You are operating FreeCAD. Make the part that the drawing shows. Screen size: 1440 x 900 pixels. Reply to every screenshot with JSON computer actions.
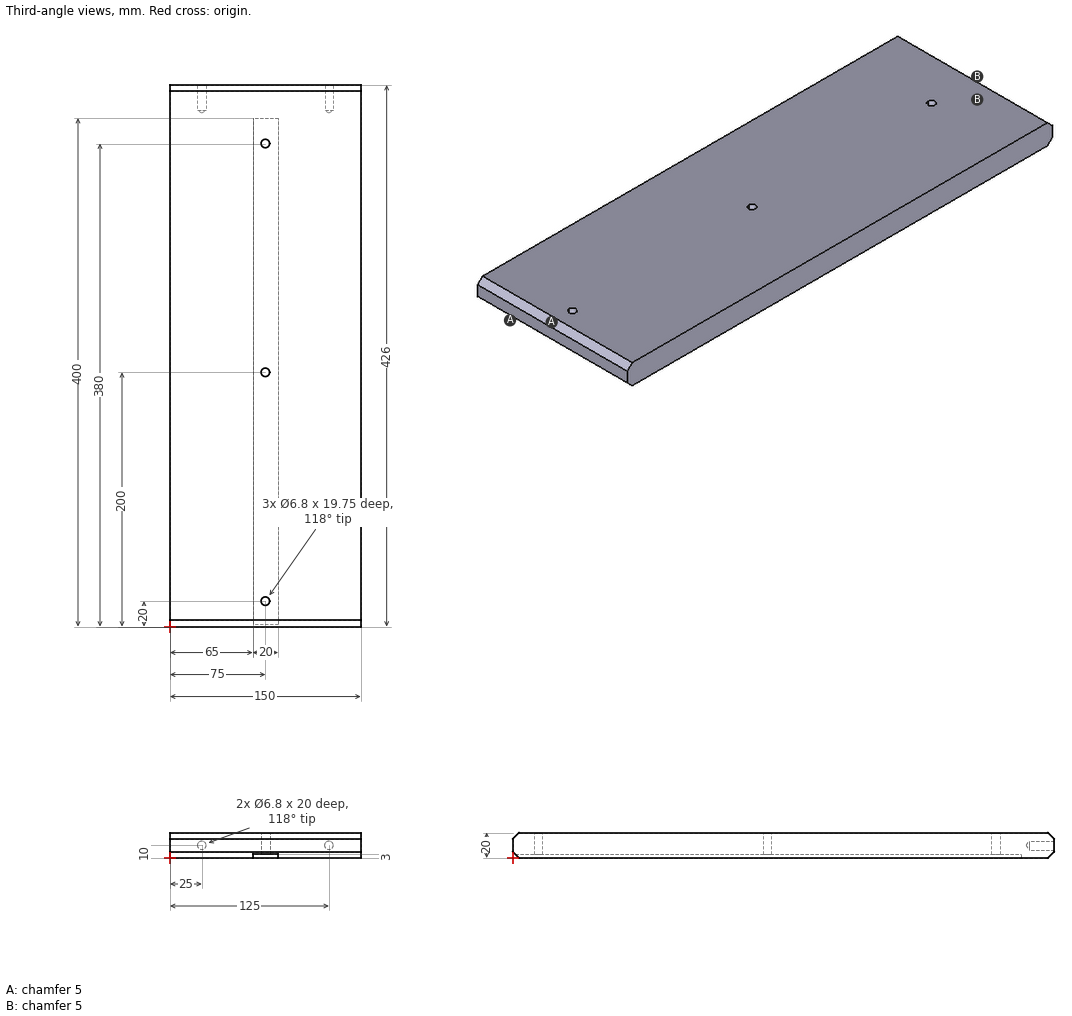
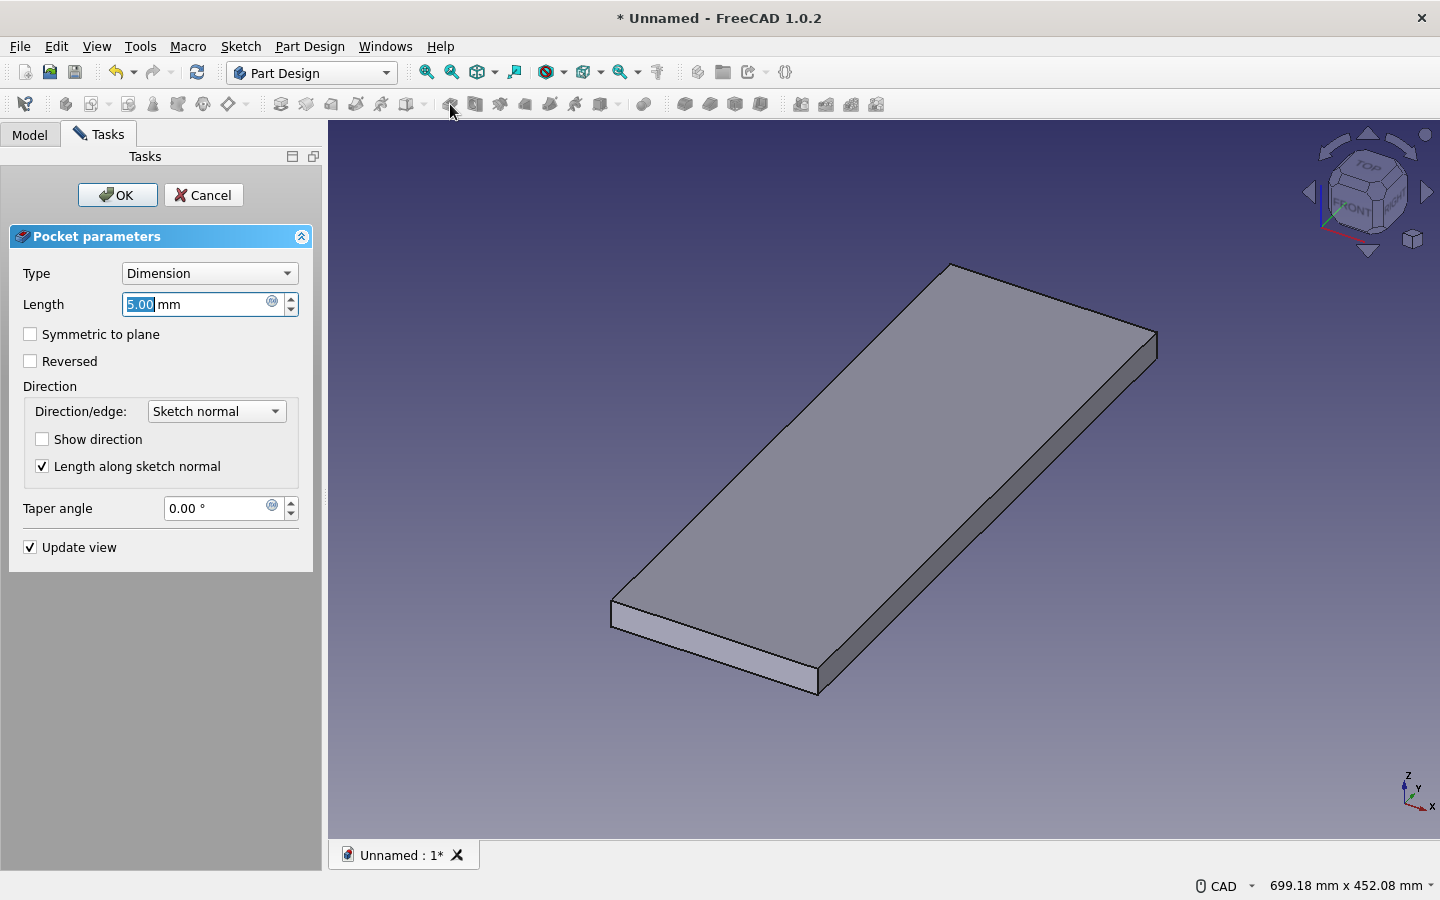
{"action": "type", "text": "3"}
{"action": "key", "text": "Tab"}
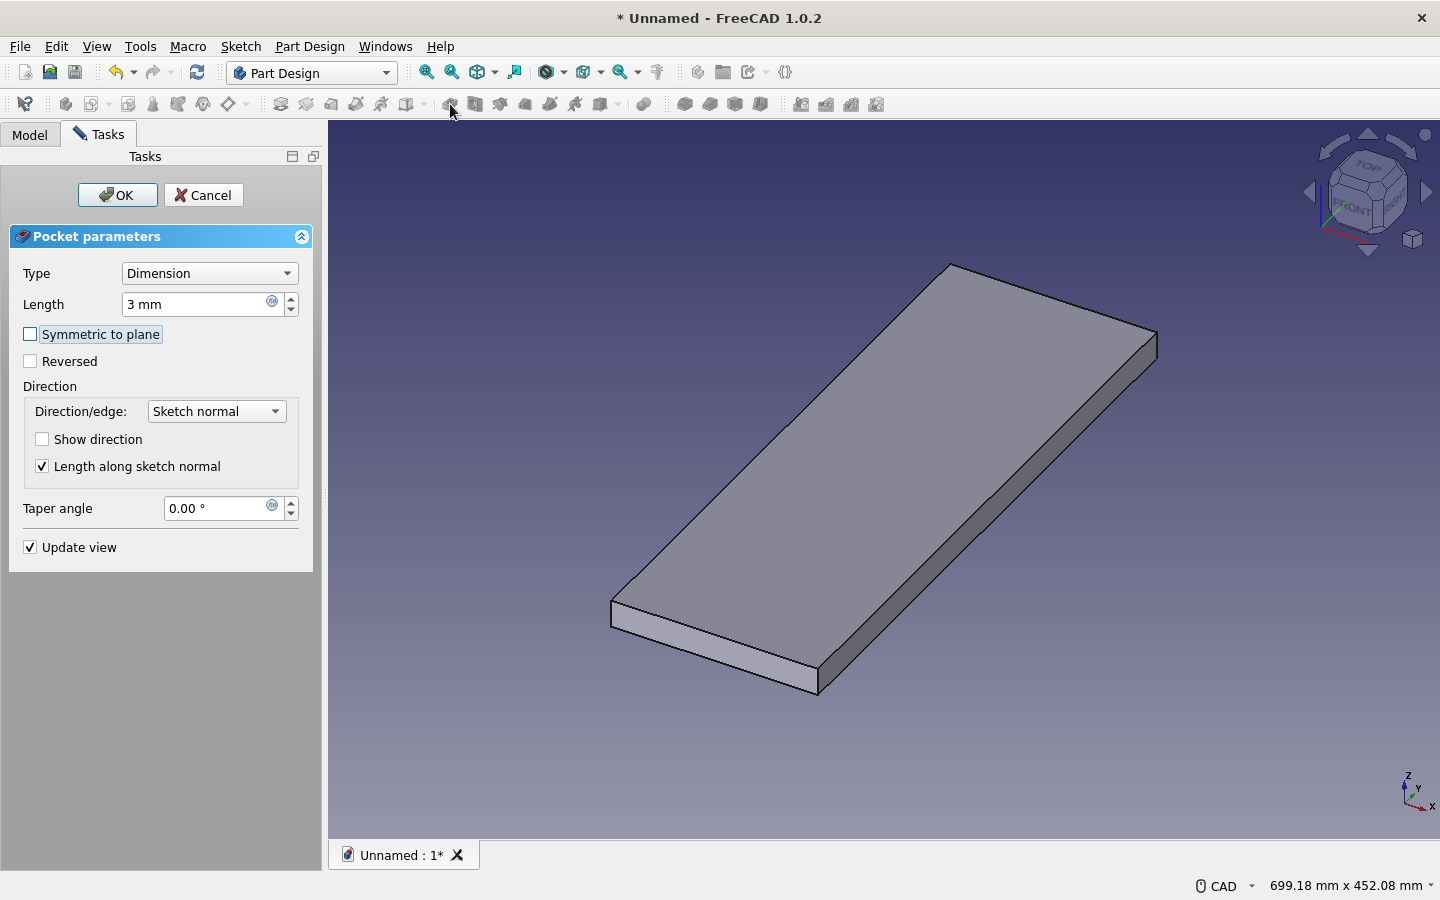
{"action": "left_click", "coordinate": [31, 361]}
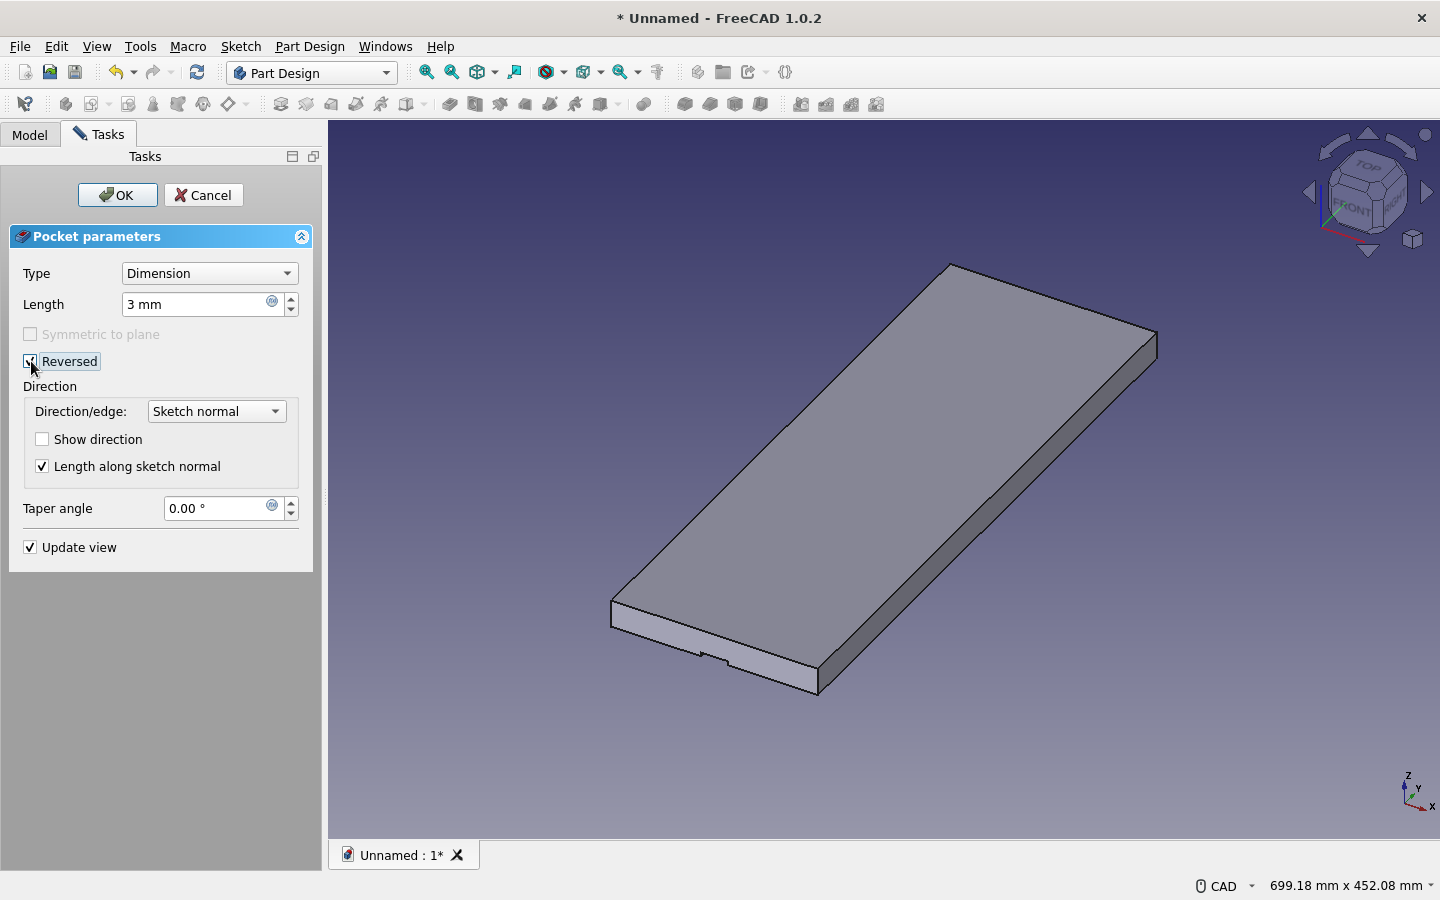
{"action": "left_click", "coordinate": [118, 195]}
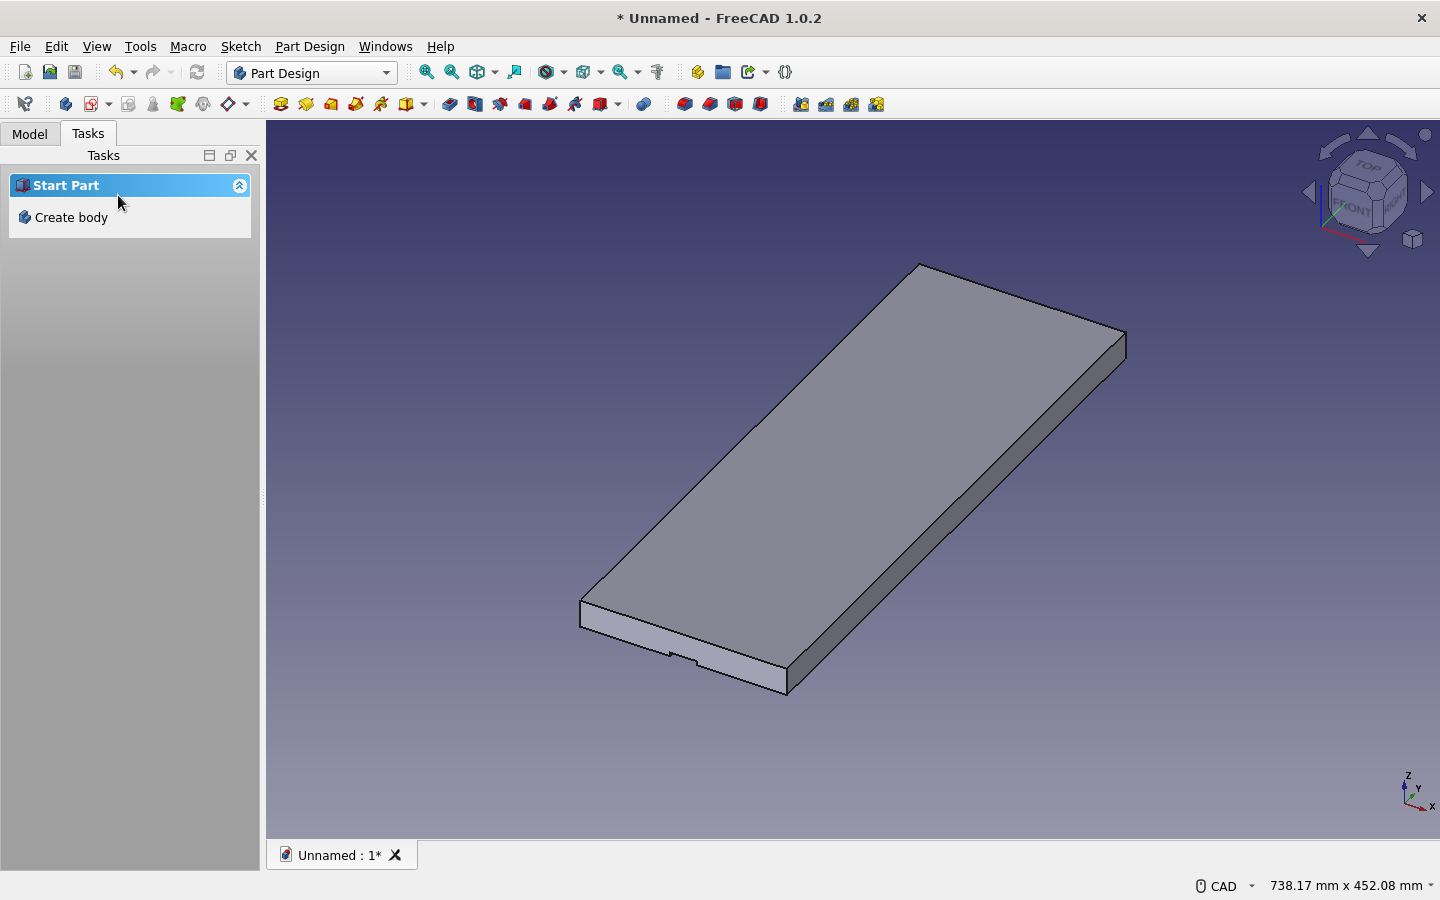
{"action": "key", "text": "5"}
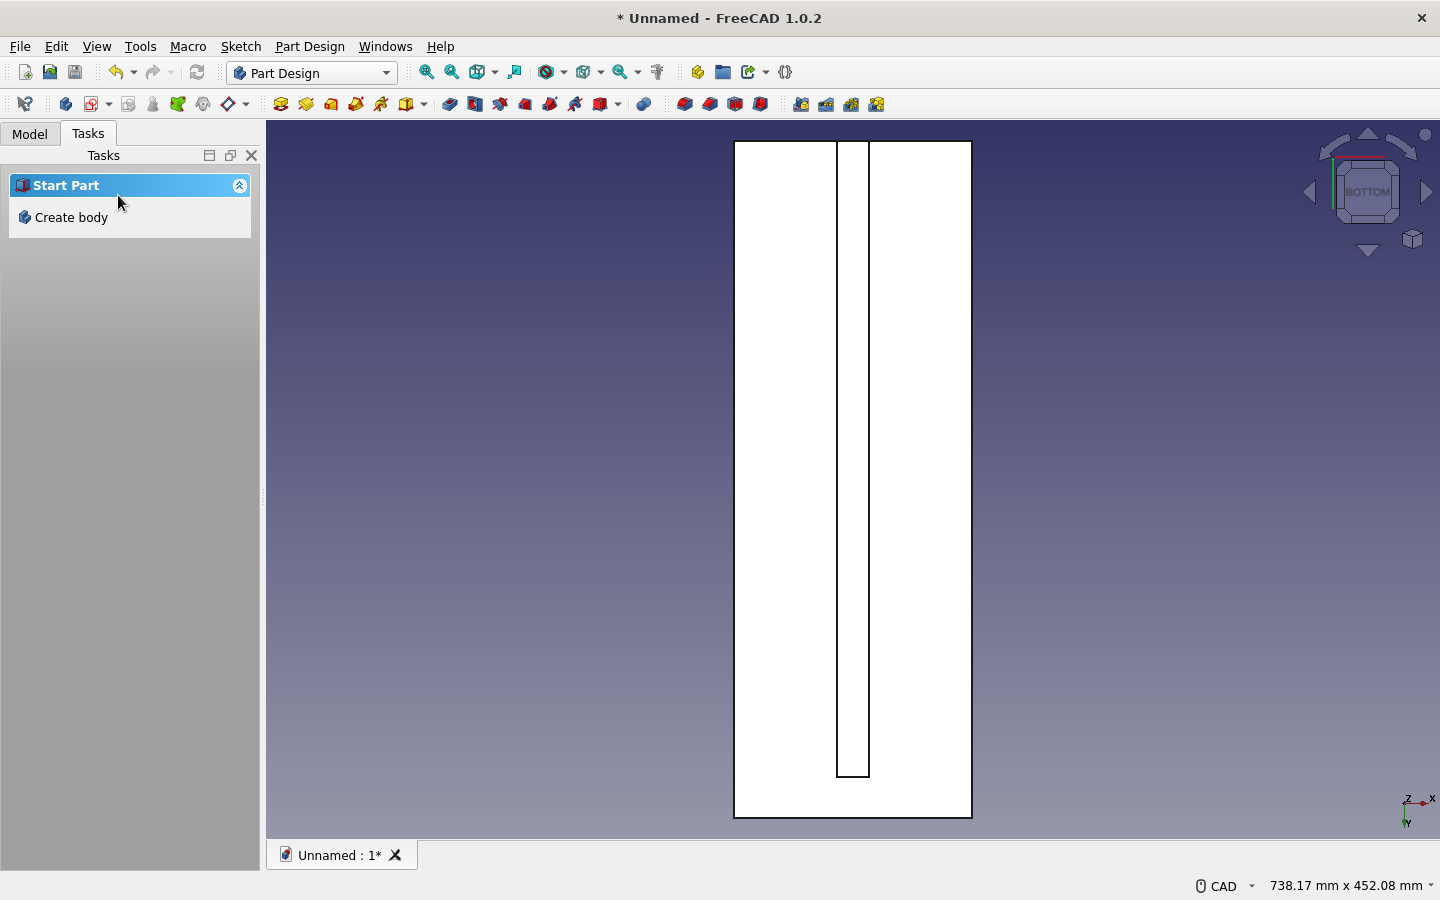
{"action": "left_click", "coordinate": [853, 730]}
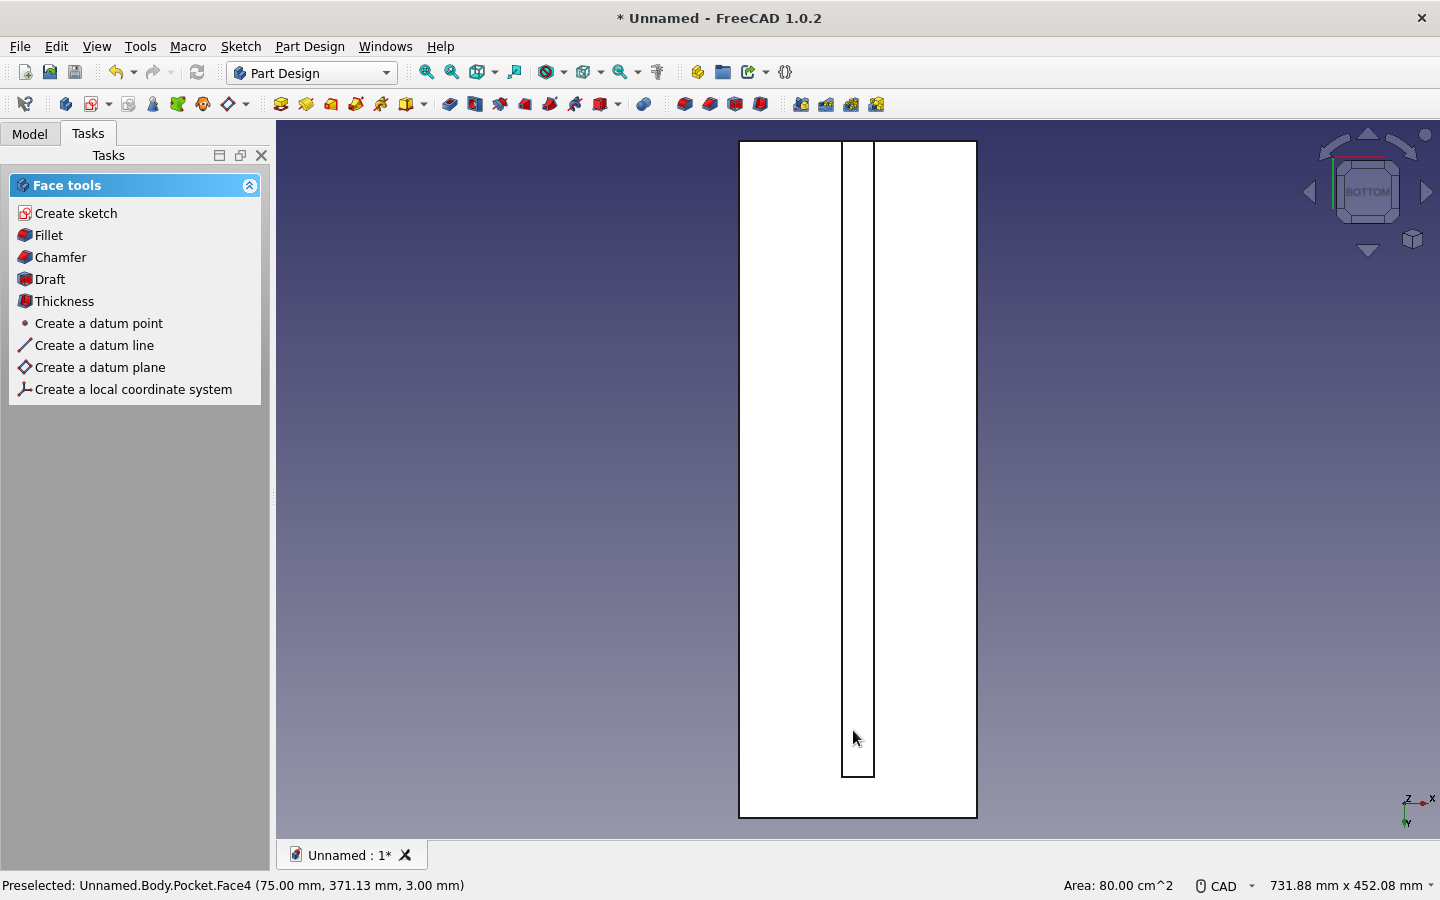
{"action": "left_click", "coordinate": [90, 104]}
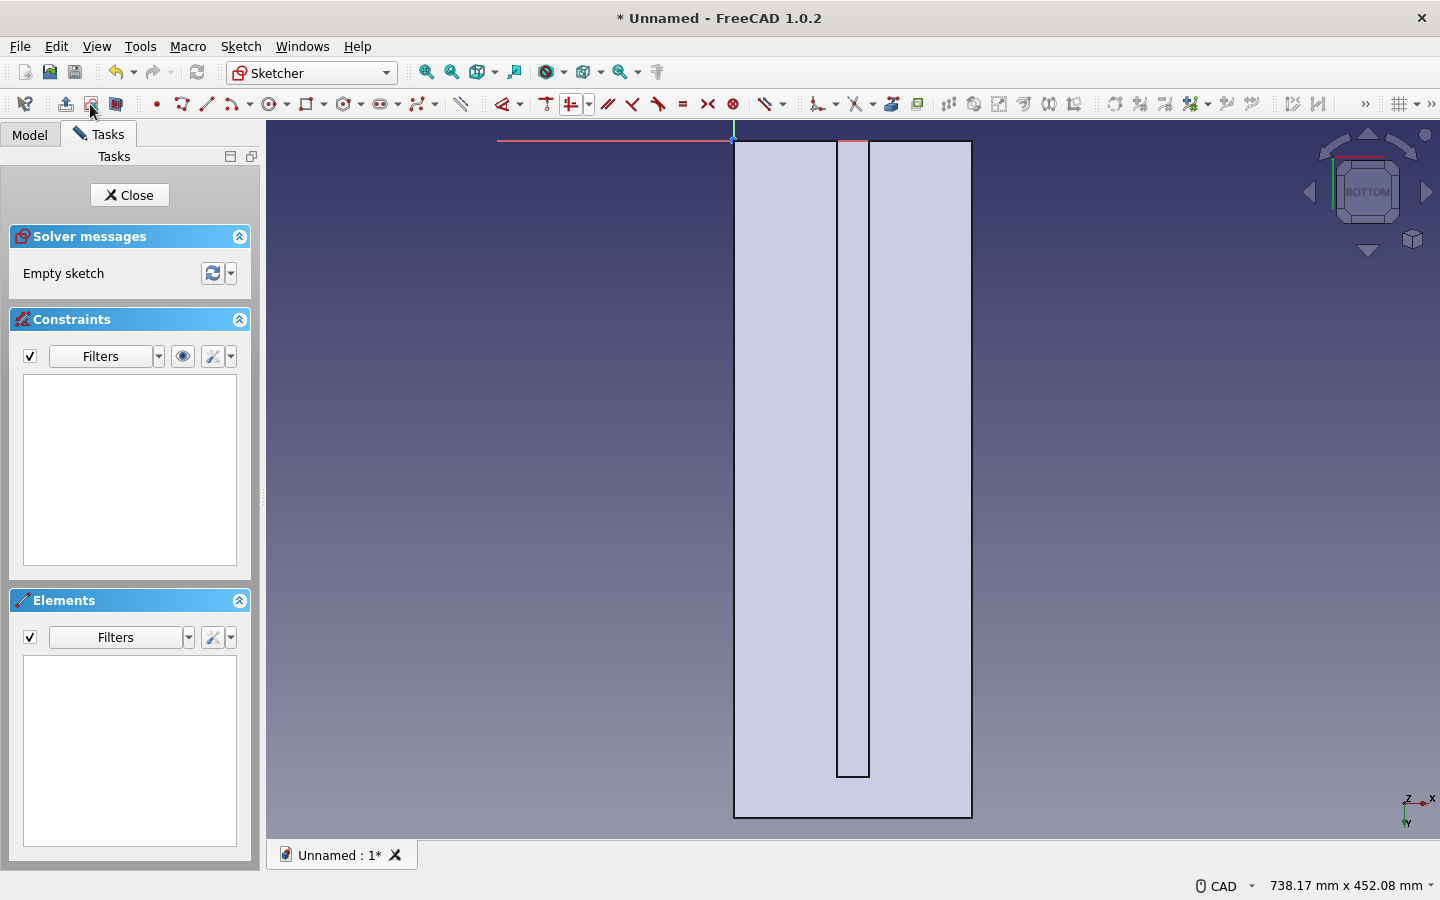
{"action": "key", "text": "q s"}